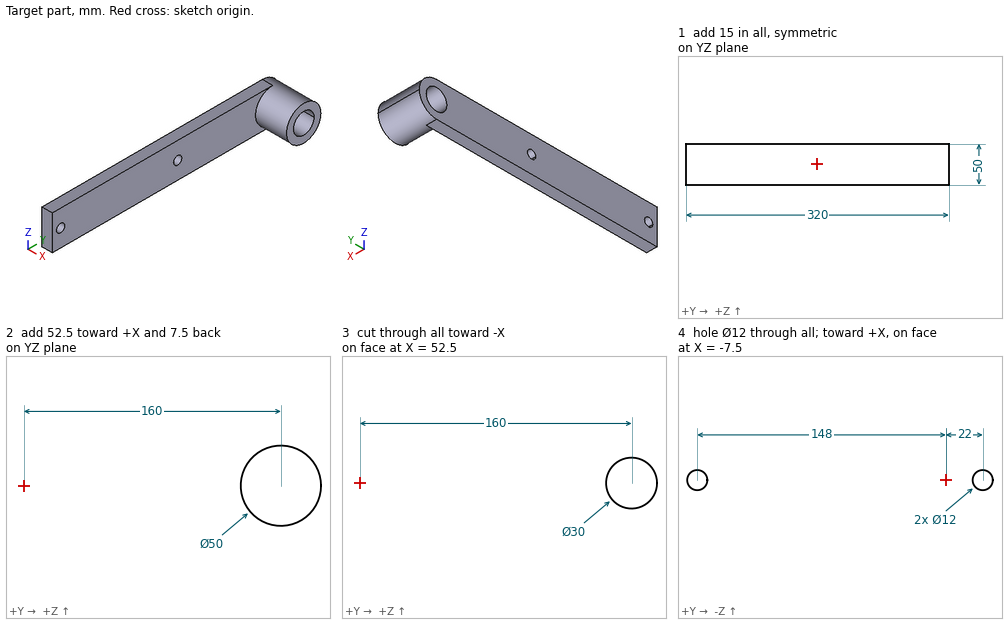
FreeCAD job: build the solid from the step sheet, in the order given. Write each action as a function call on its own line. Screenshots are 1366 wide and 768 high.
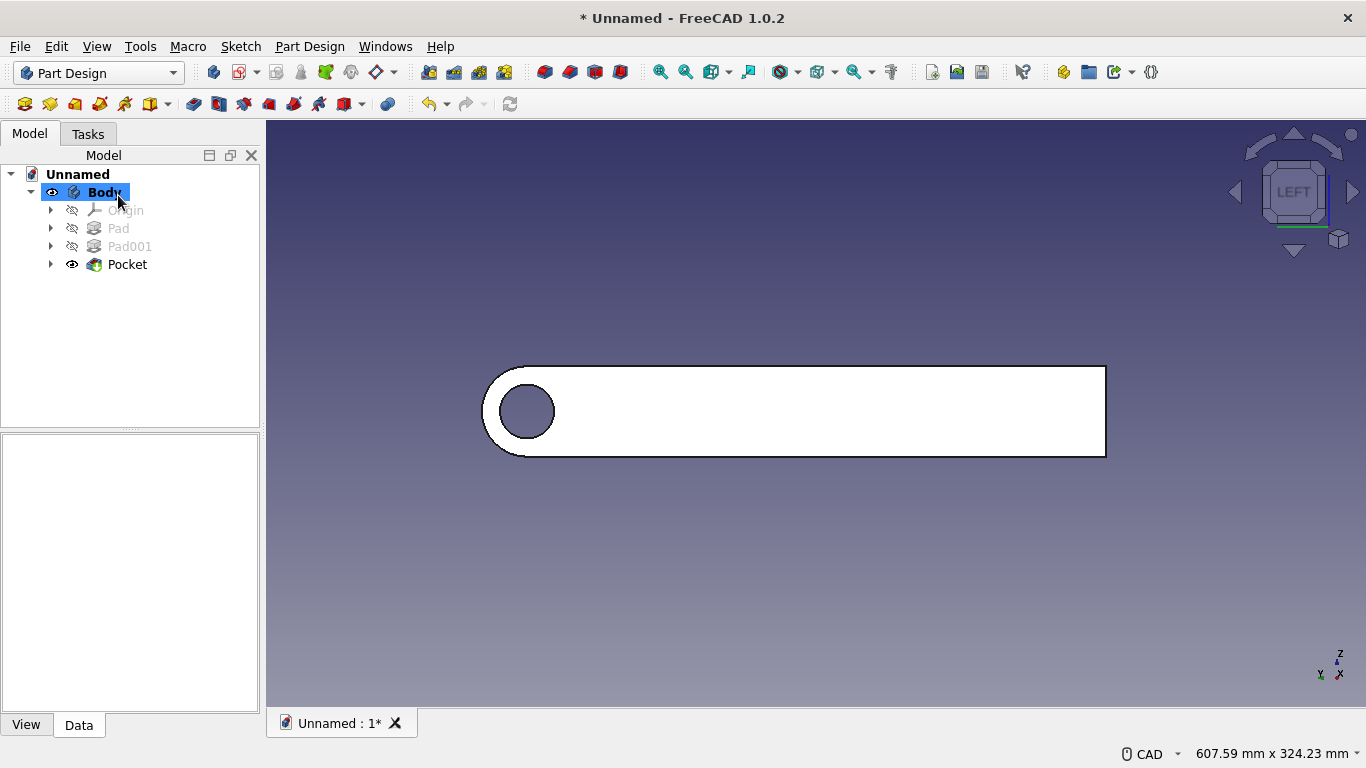
click(794, 410)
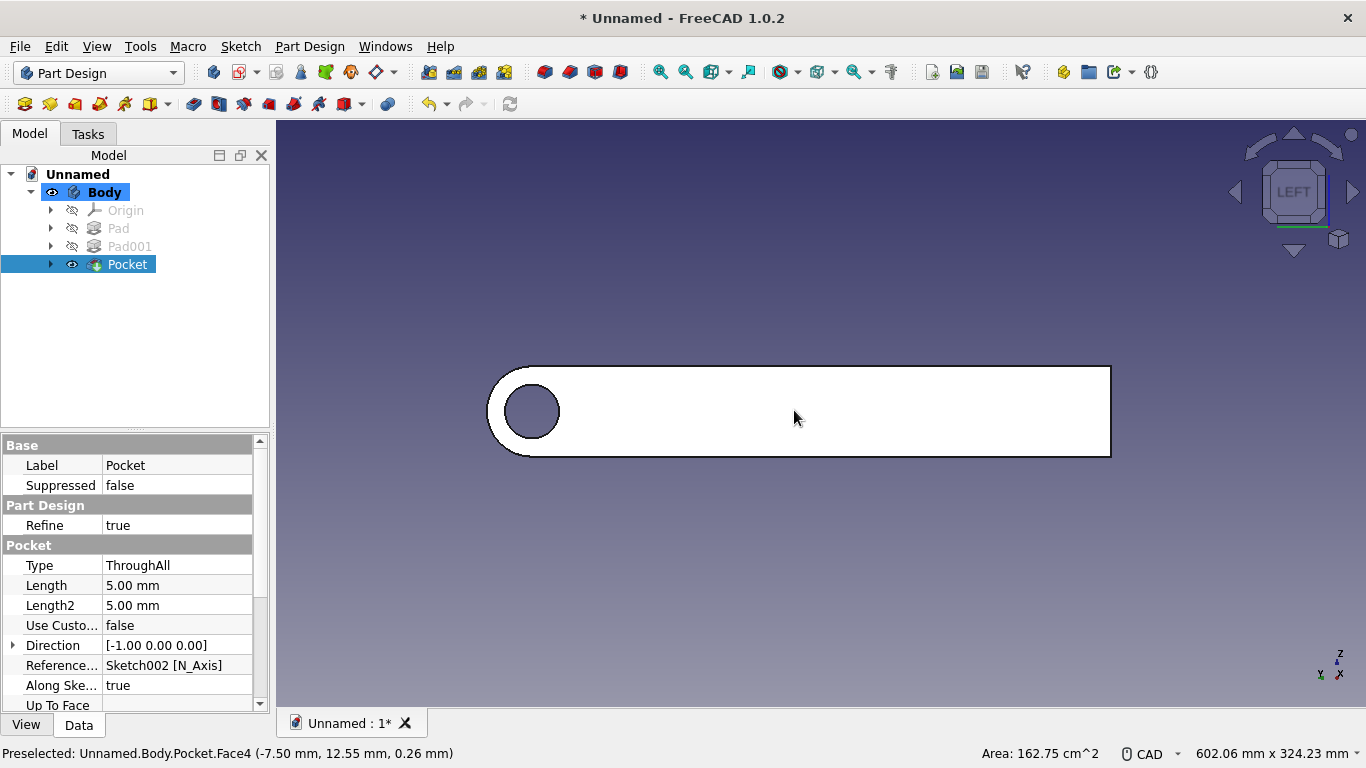
click(238, 72)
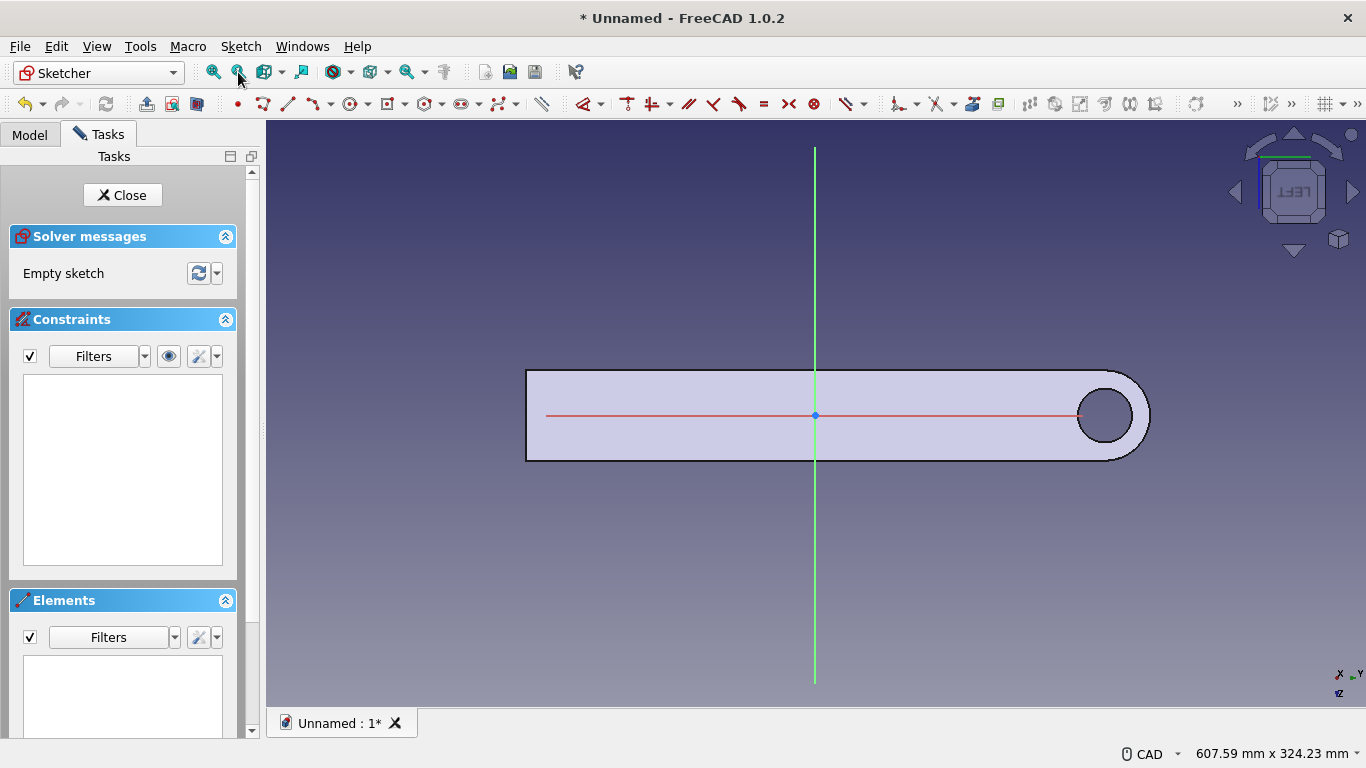
scroll(645, 418, up, 3)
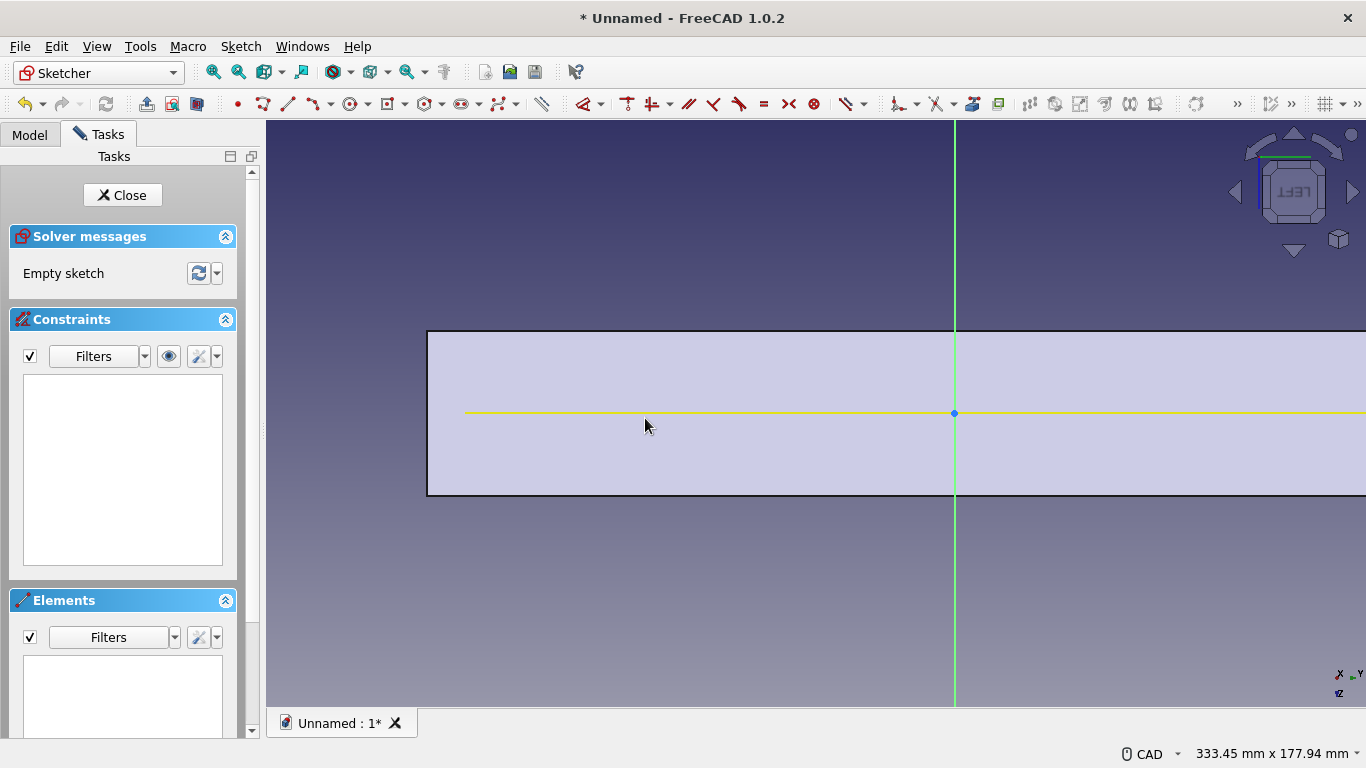
click(350, 104)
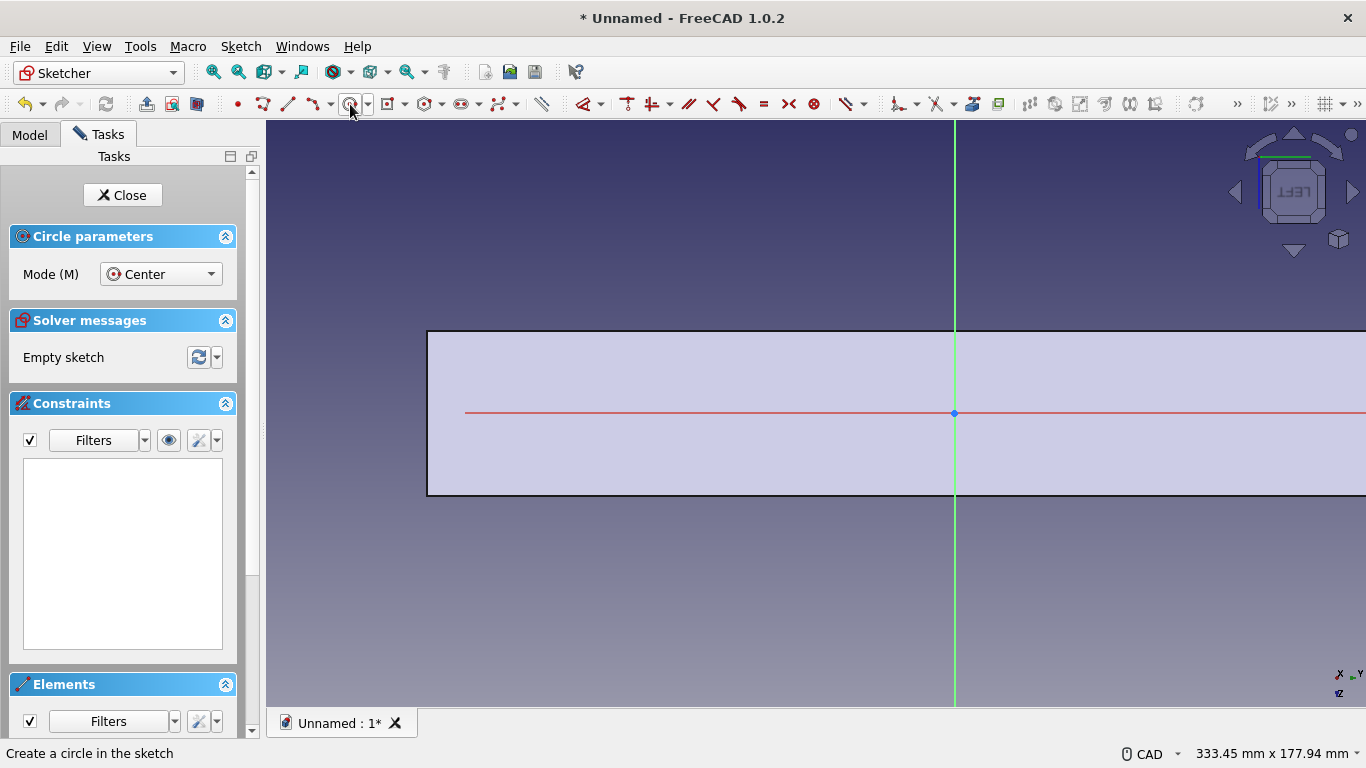
click(1028, 413)
click(1034, 394)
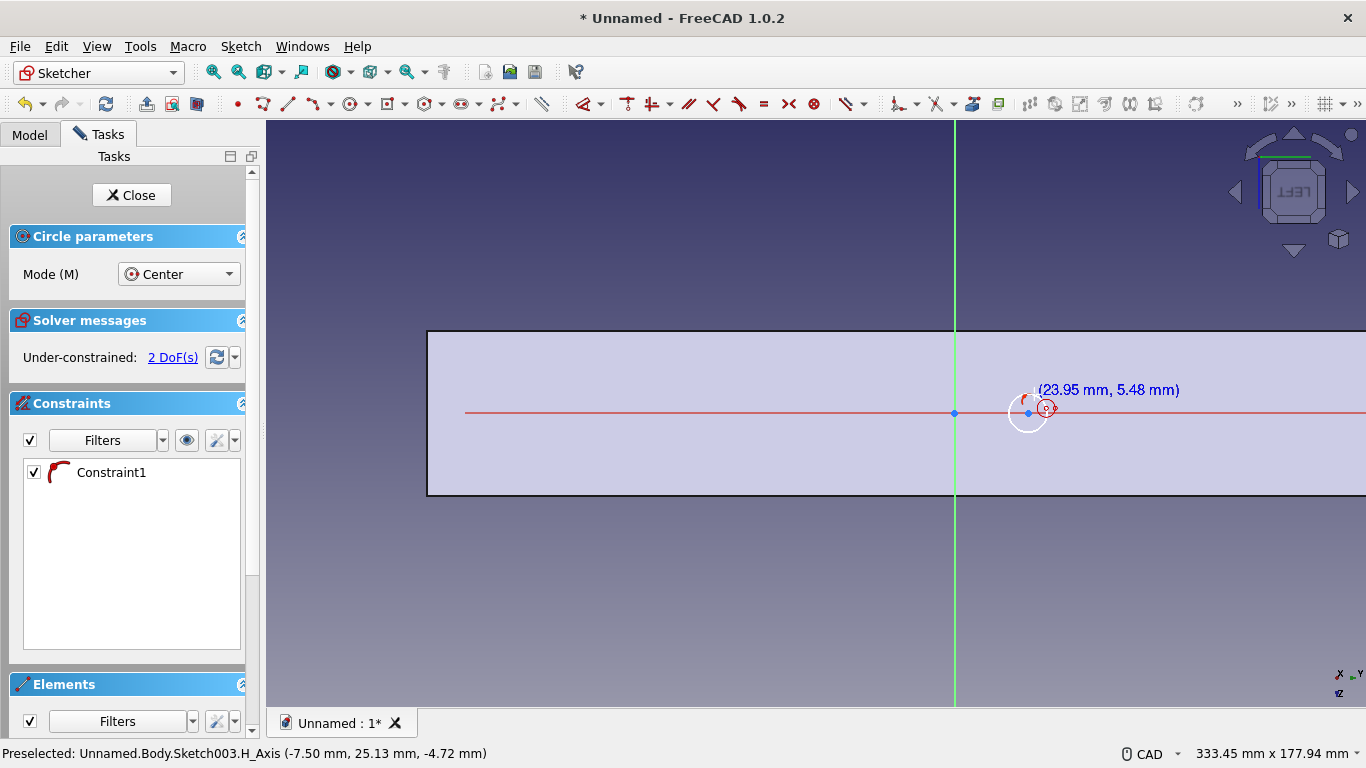
click(467, 413)
click(474, 394)
key(Escape)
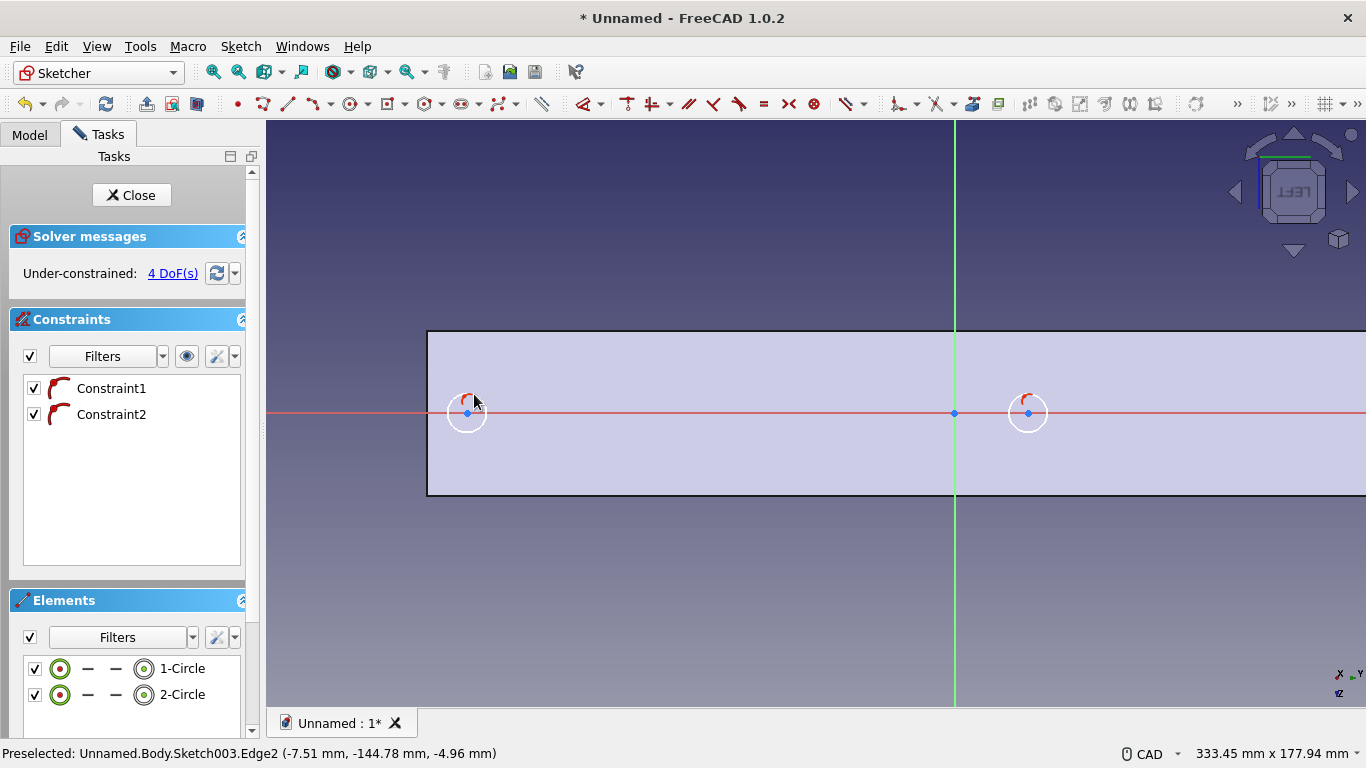
click(1041, 400)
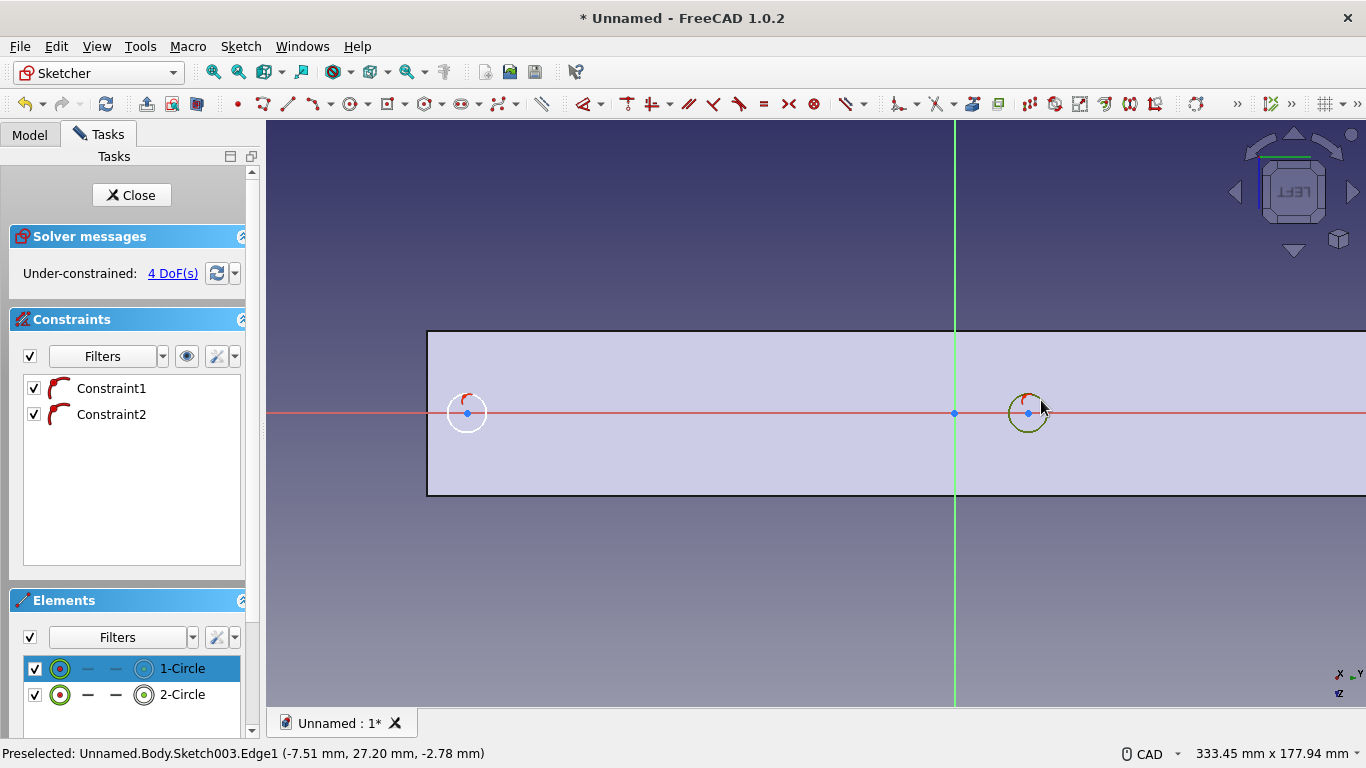
click(481, 399)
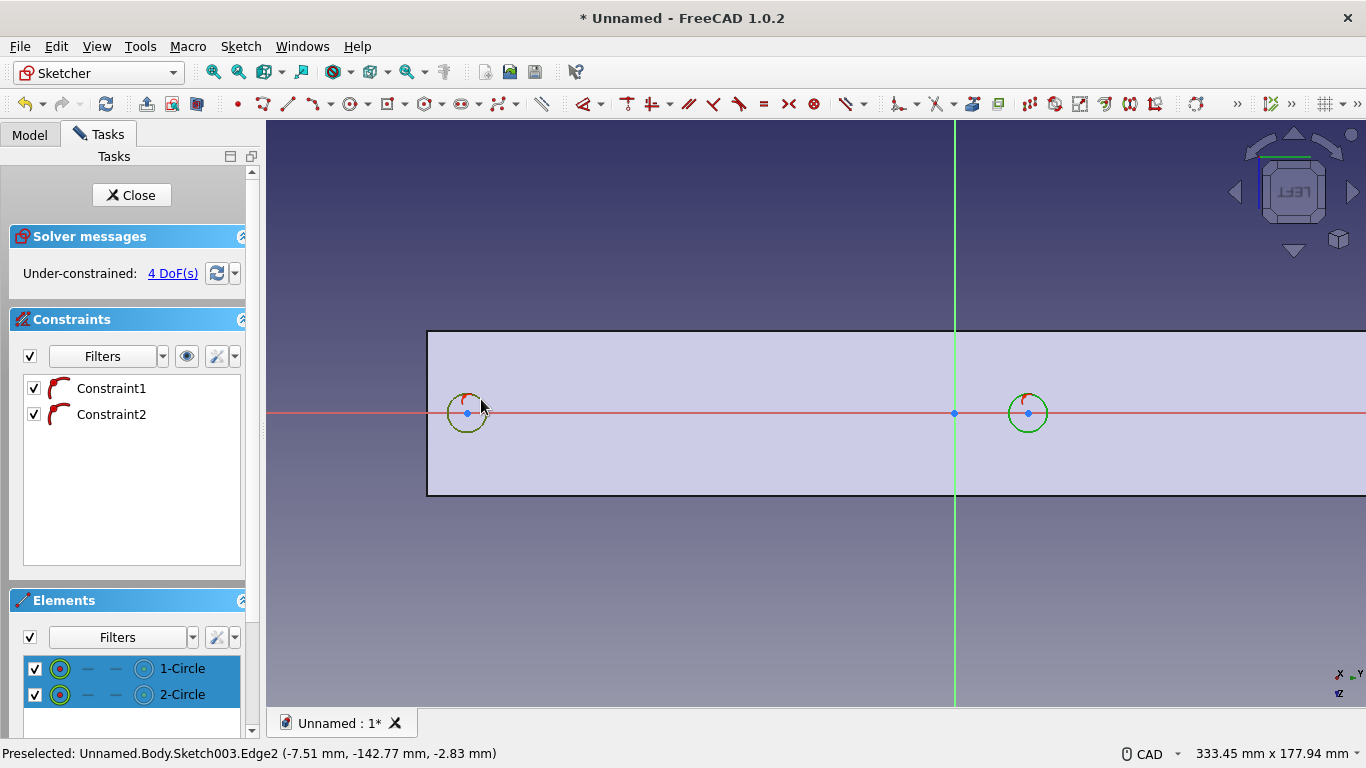
click(764, 104)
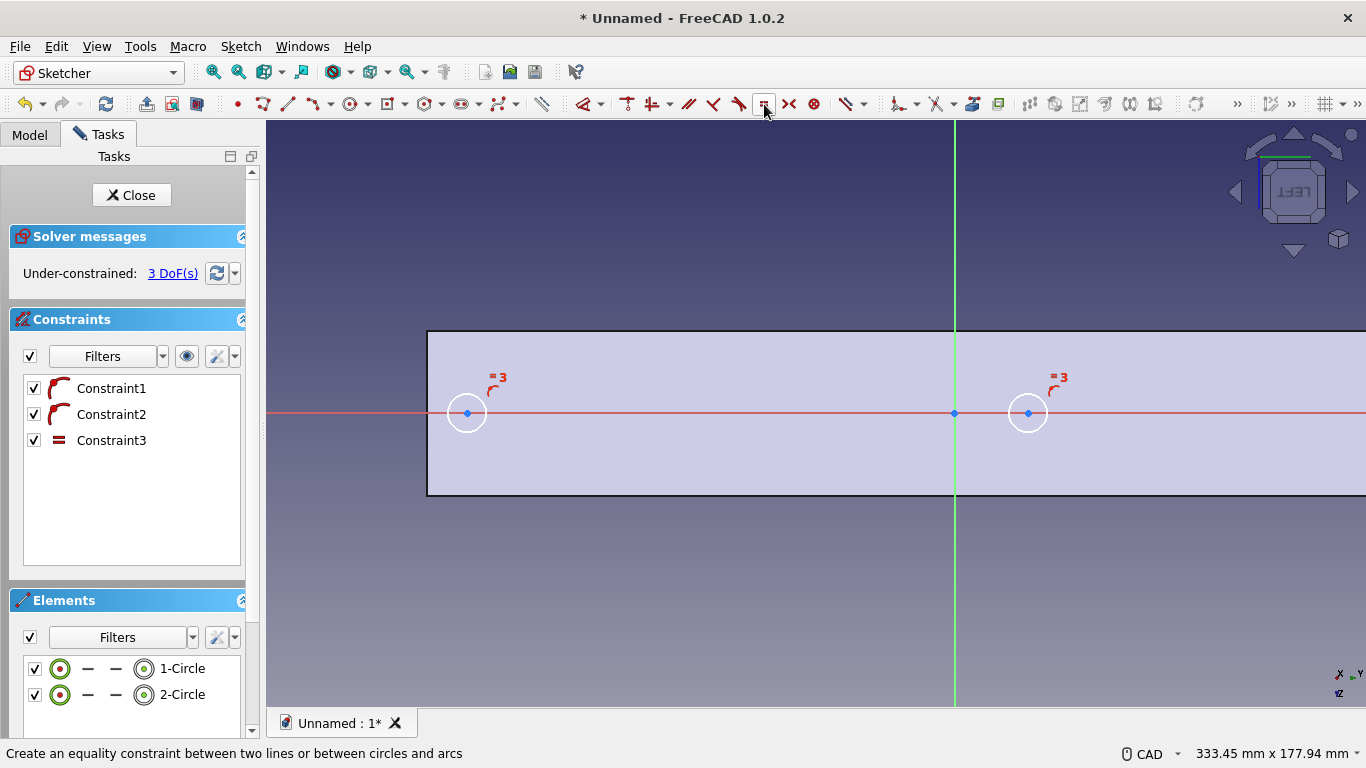
click(582, 104)